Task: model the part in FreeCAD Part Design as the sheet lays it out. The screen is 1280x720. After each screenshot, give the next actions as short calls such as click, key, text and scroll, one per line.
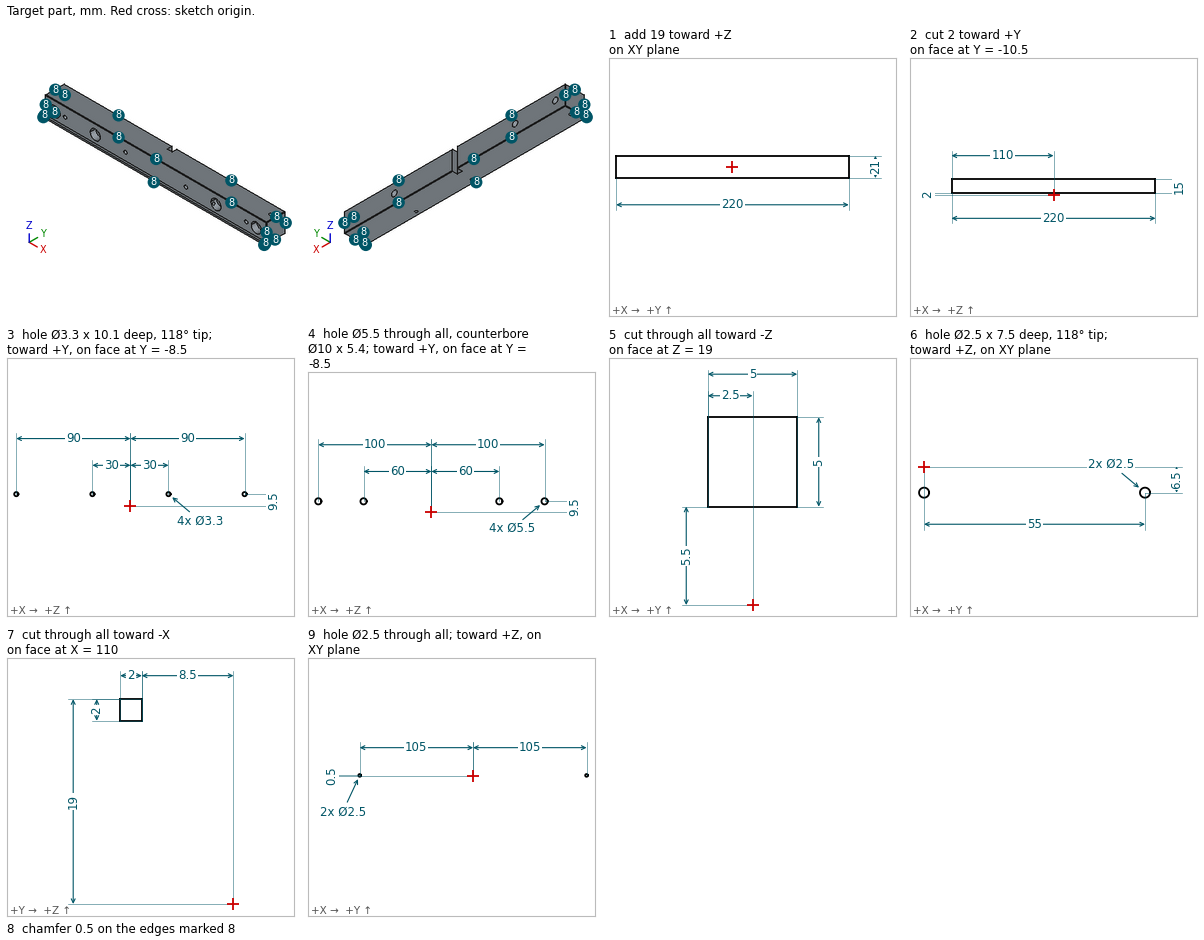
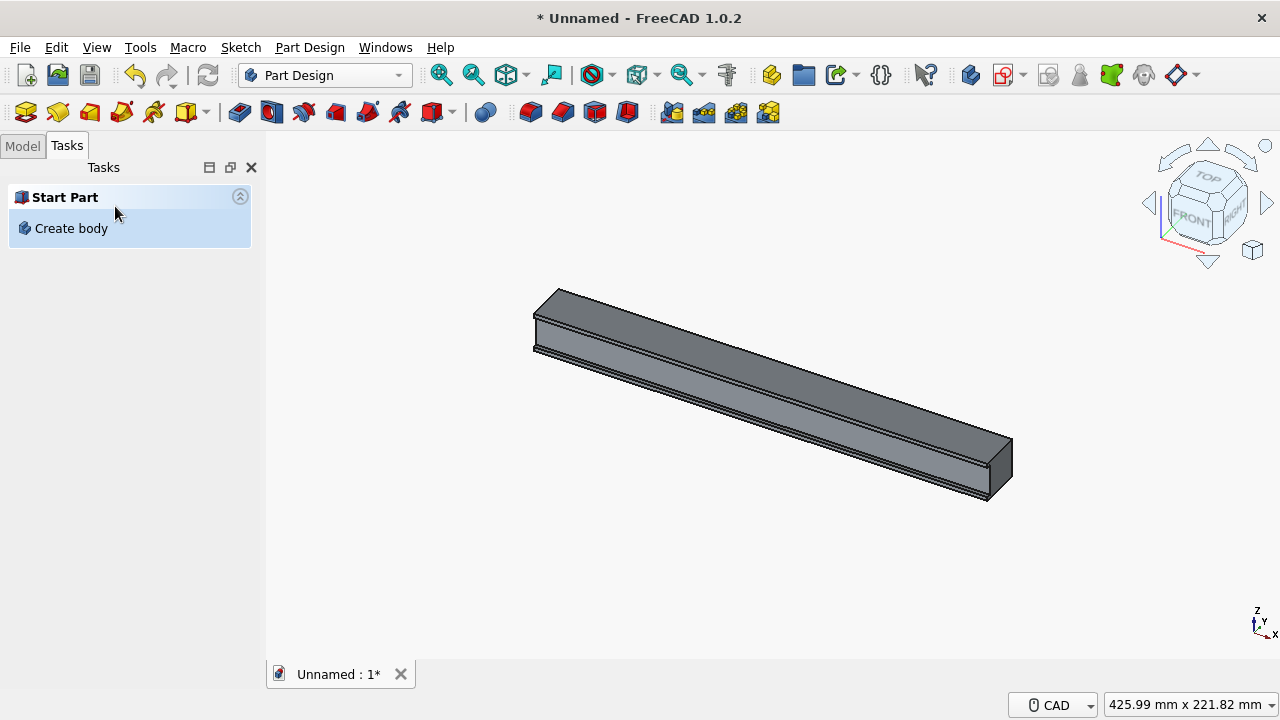
click(957, 468)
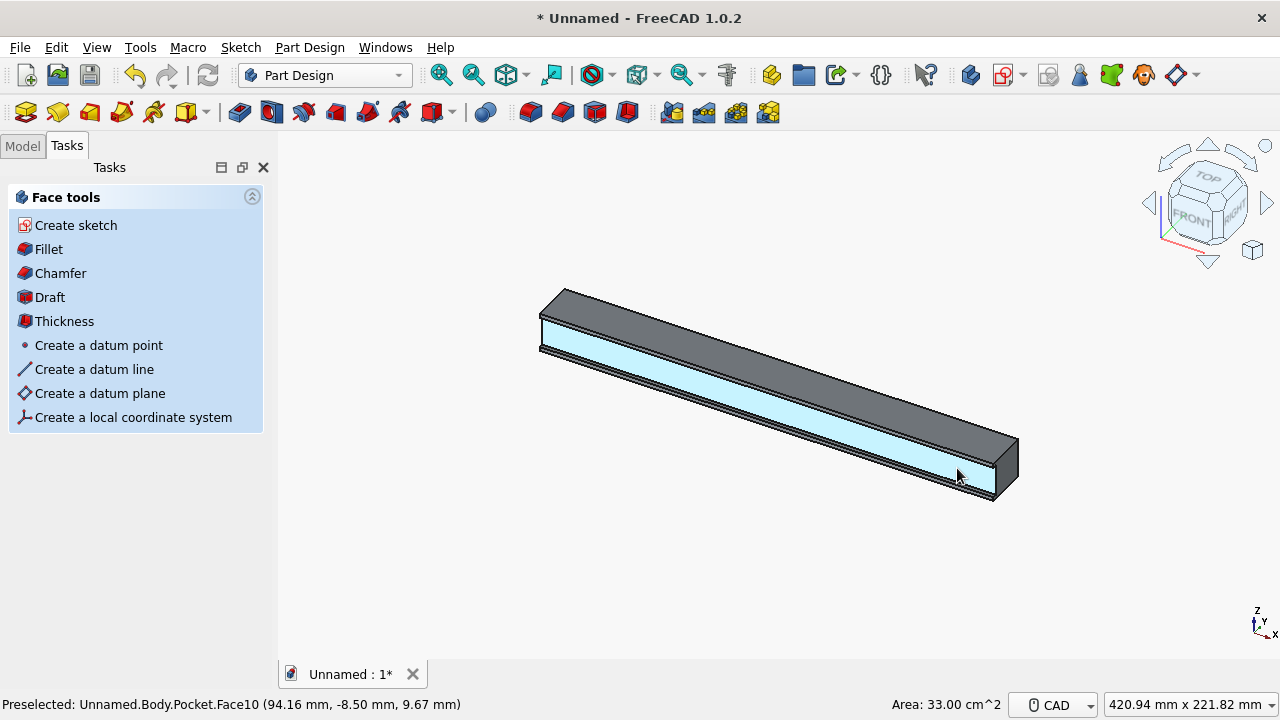
click(1004, 76)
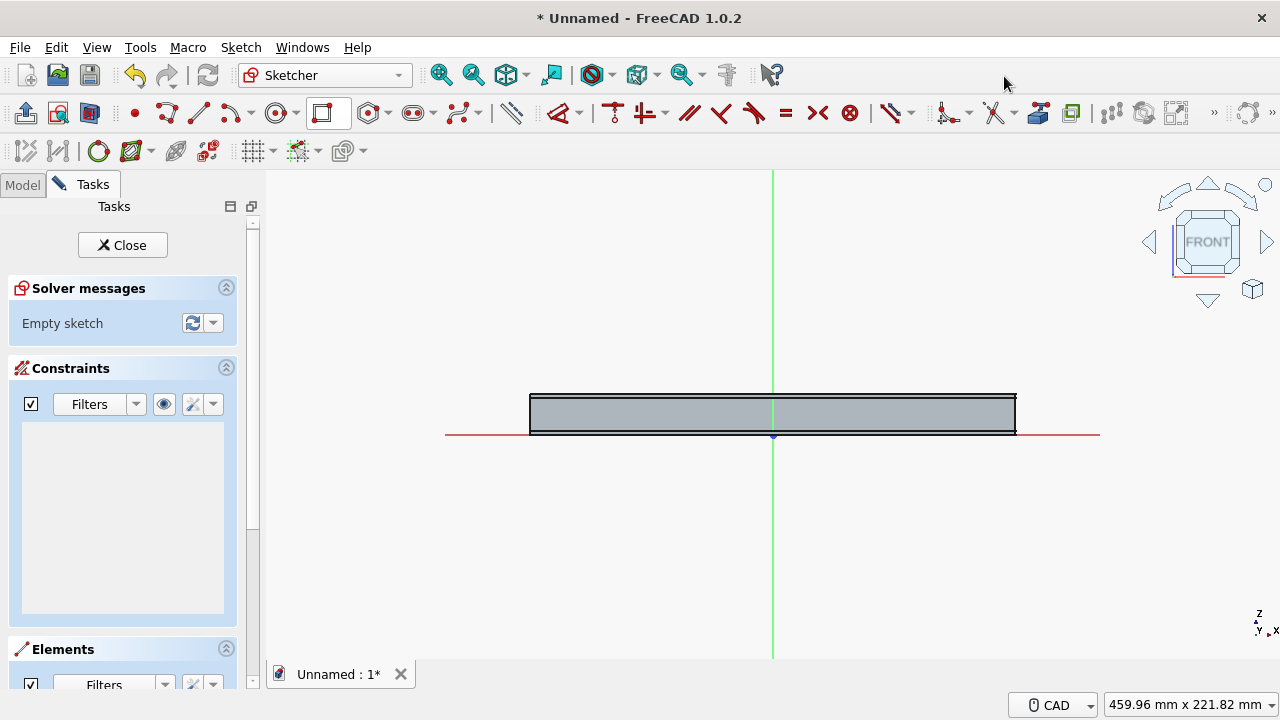
scroll(912, 441, up, 2)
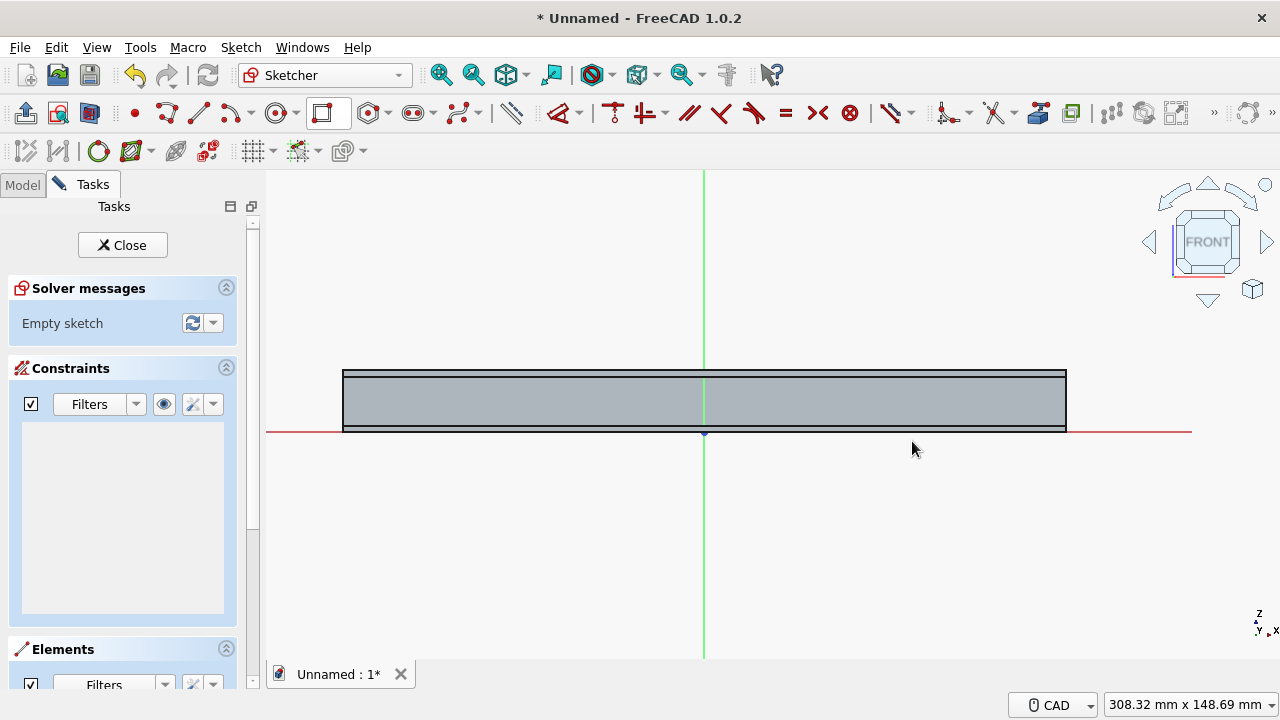
click(276, 114)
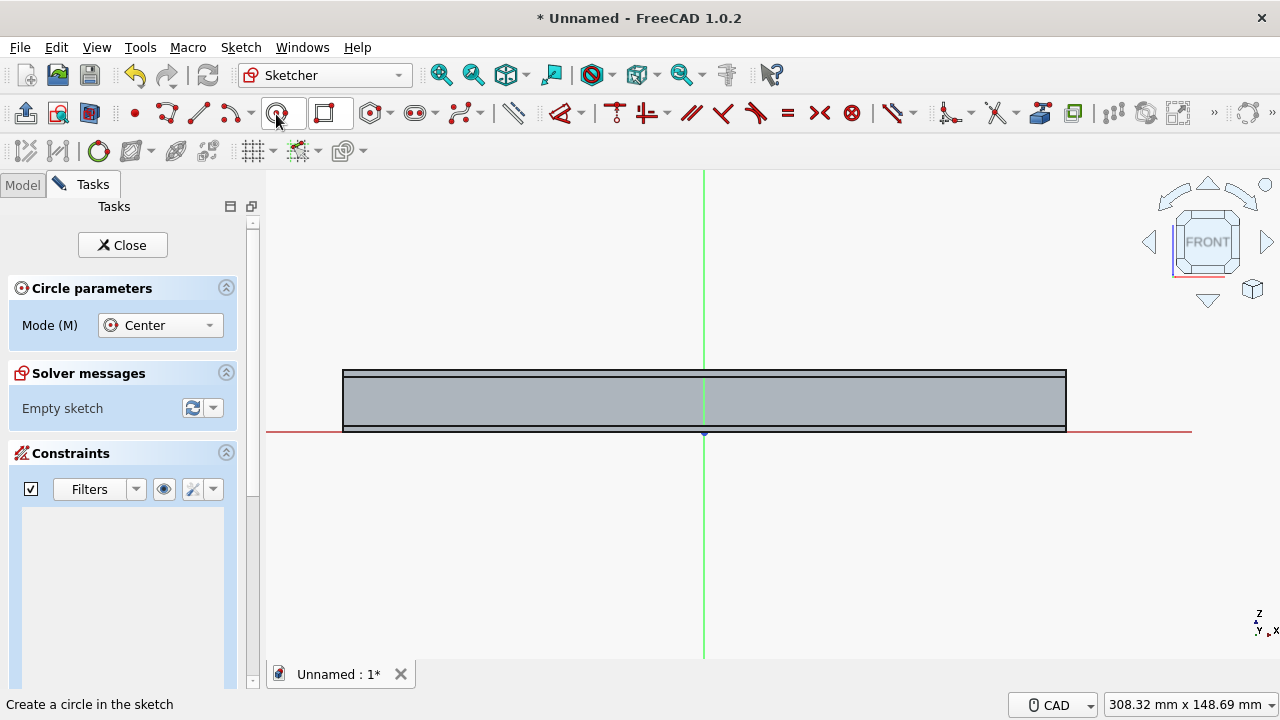
scroll(1000, 401, up, 8)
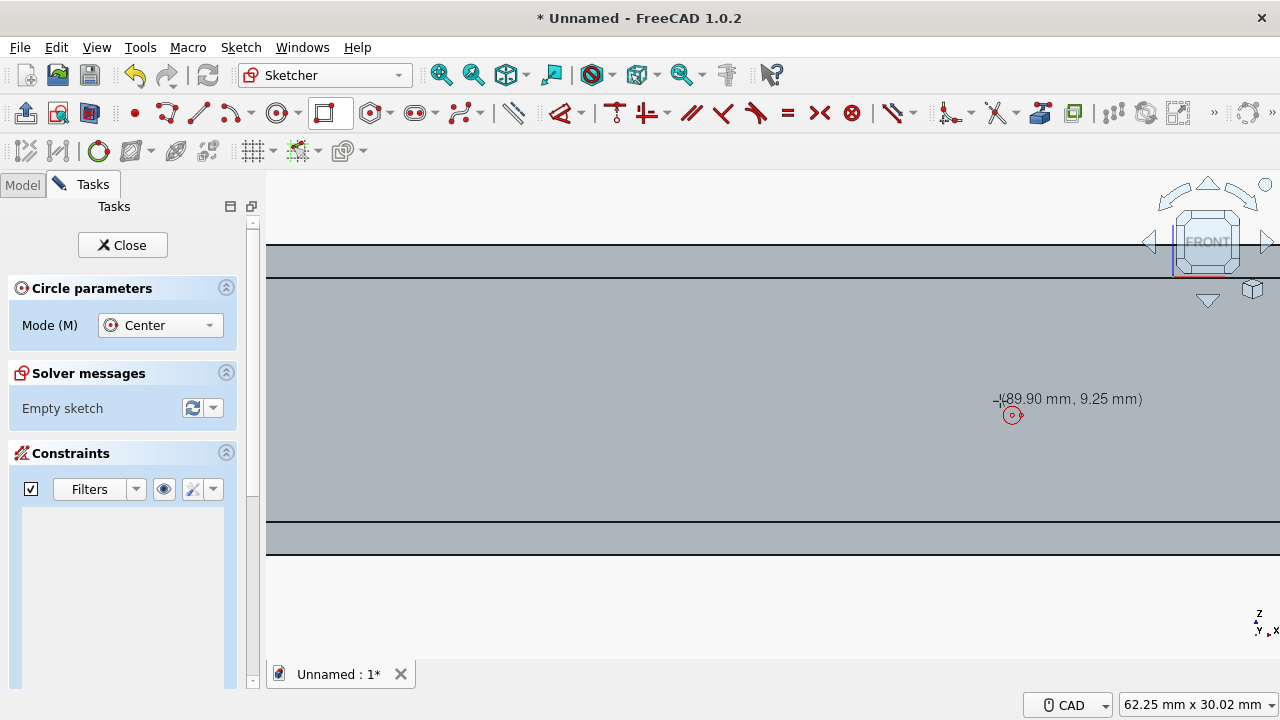
scroll(1001, 402, down, 8)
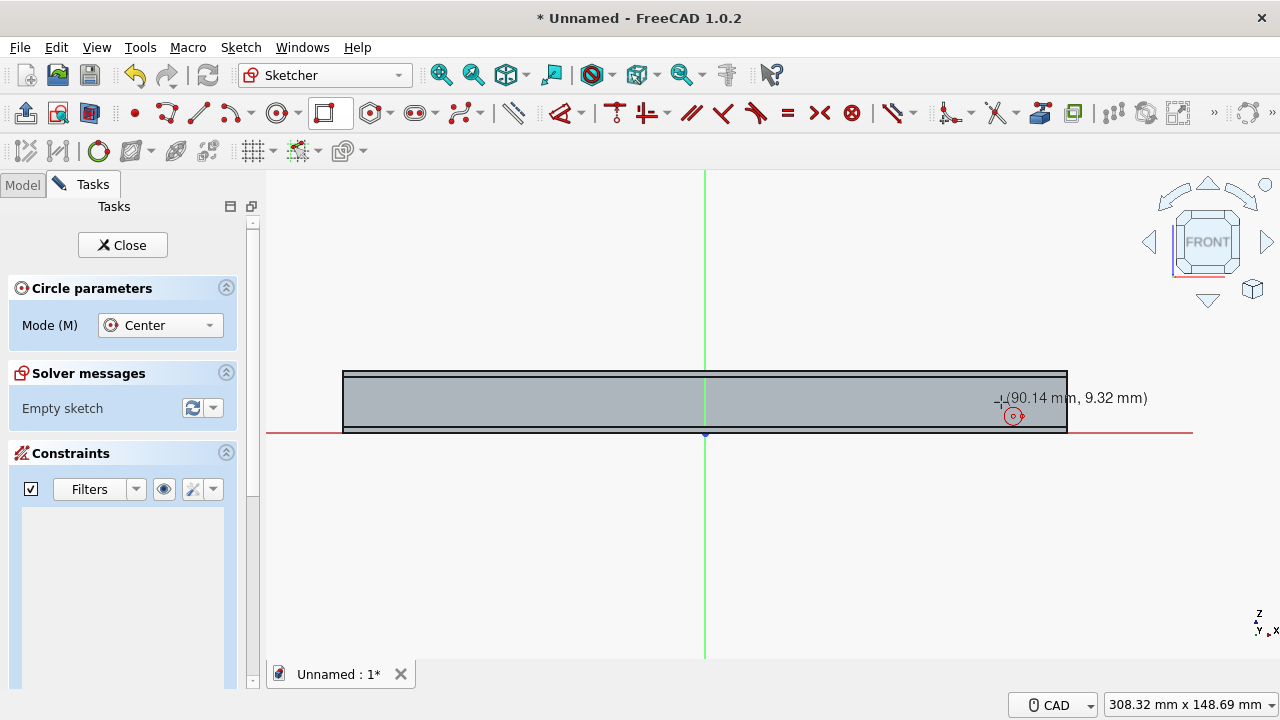
click(1001, 402)
move(1005, 398)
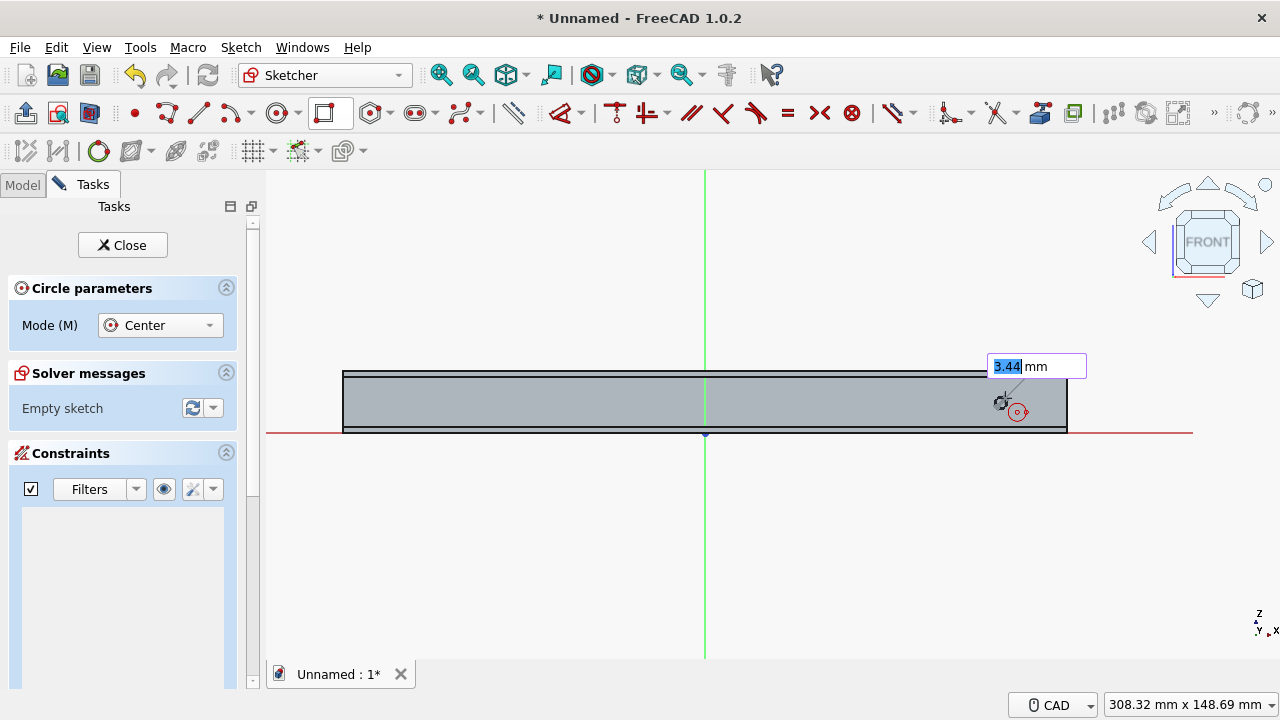
text(3.3)
key(Return)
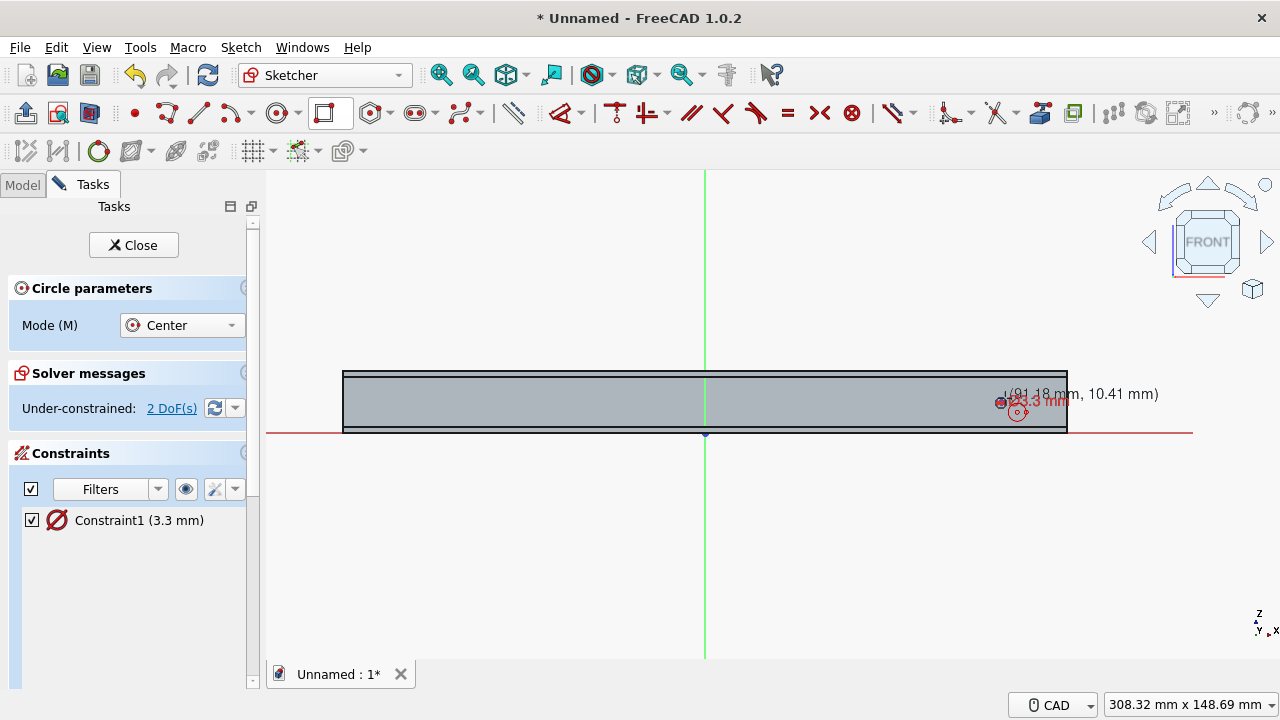
scroll(804, 402, up, 8)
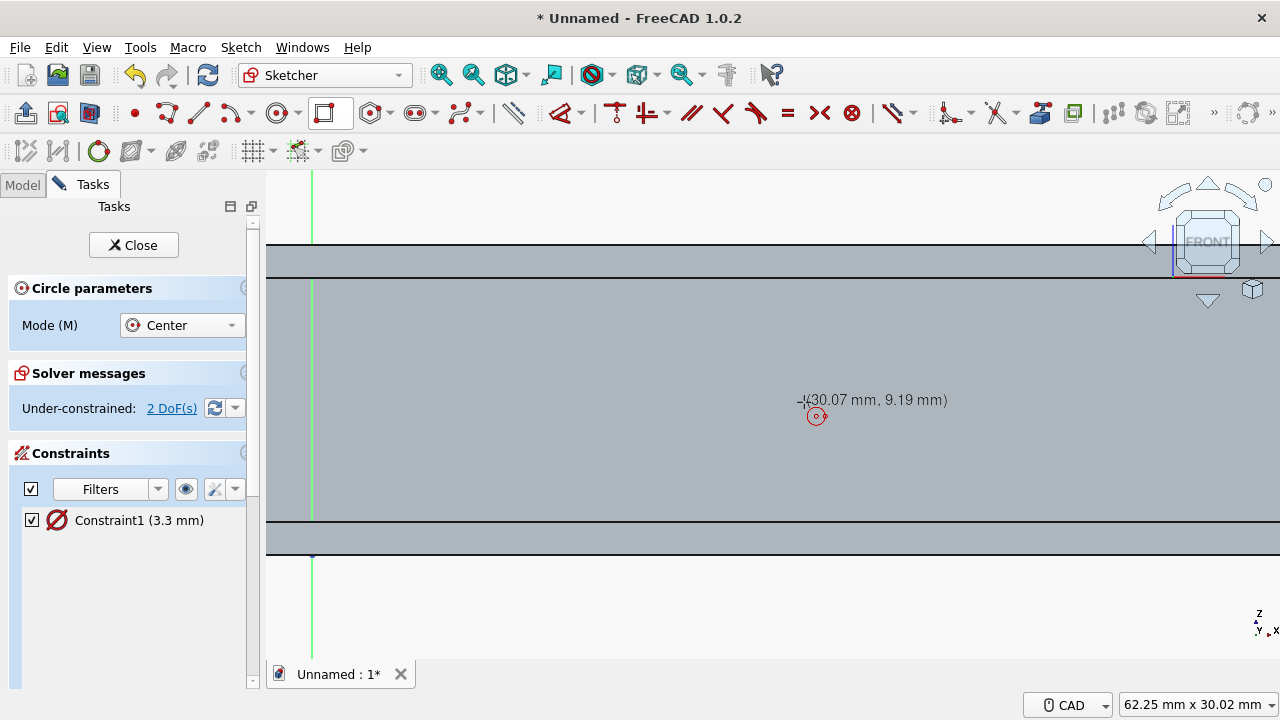
scroll(804, 402, down, 8)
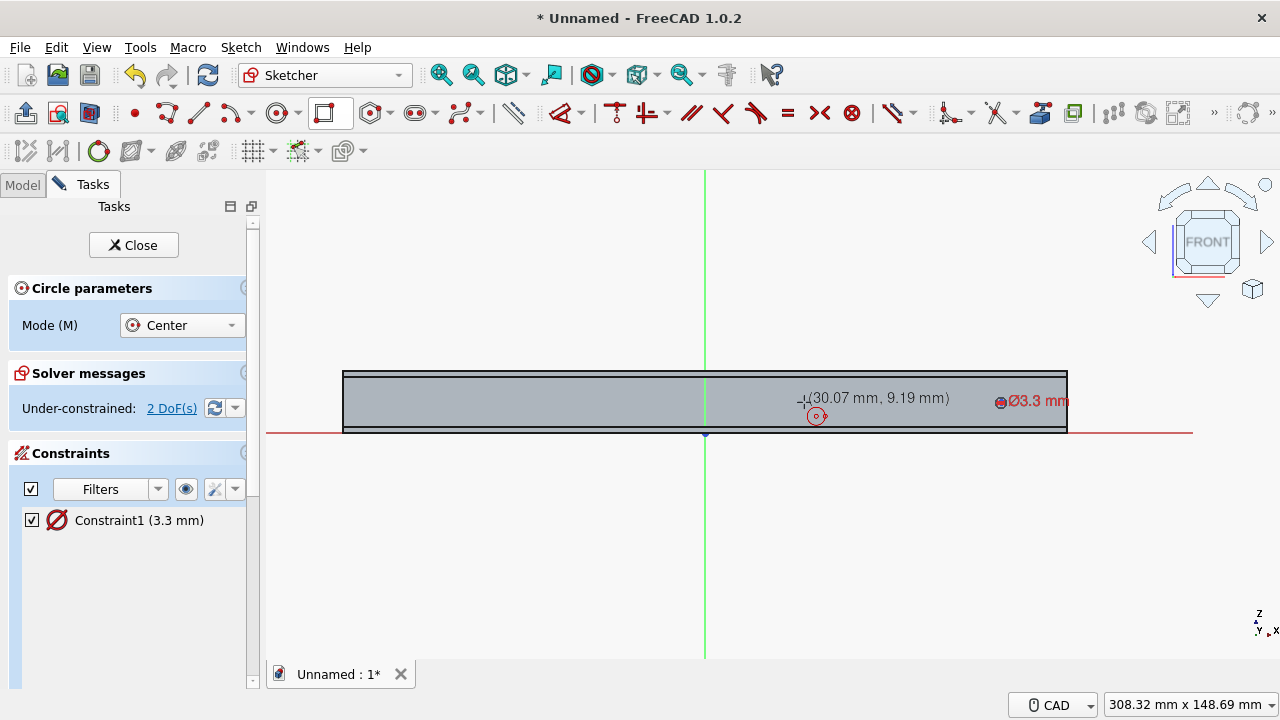
click(804, 402)
move(808, 398)